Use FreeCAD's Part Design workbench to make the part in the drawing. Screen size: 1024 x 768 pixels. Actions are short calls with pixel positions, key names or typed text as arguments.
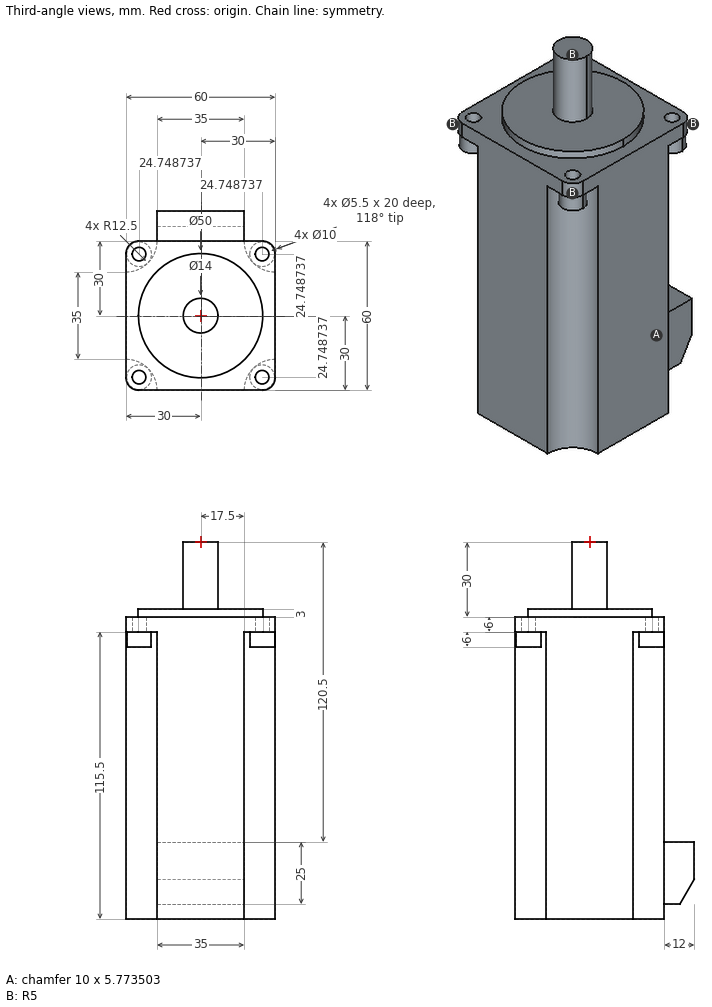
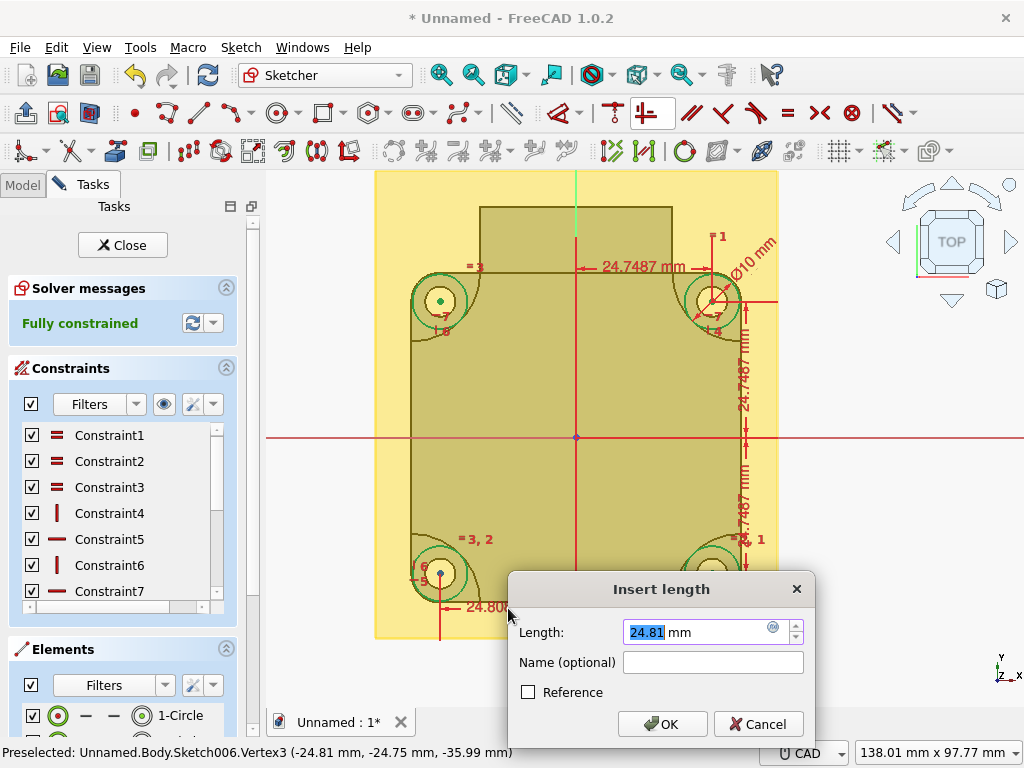
text(24.748737)
key(Return)
key(Escape)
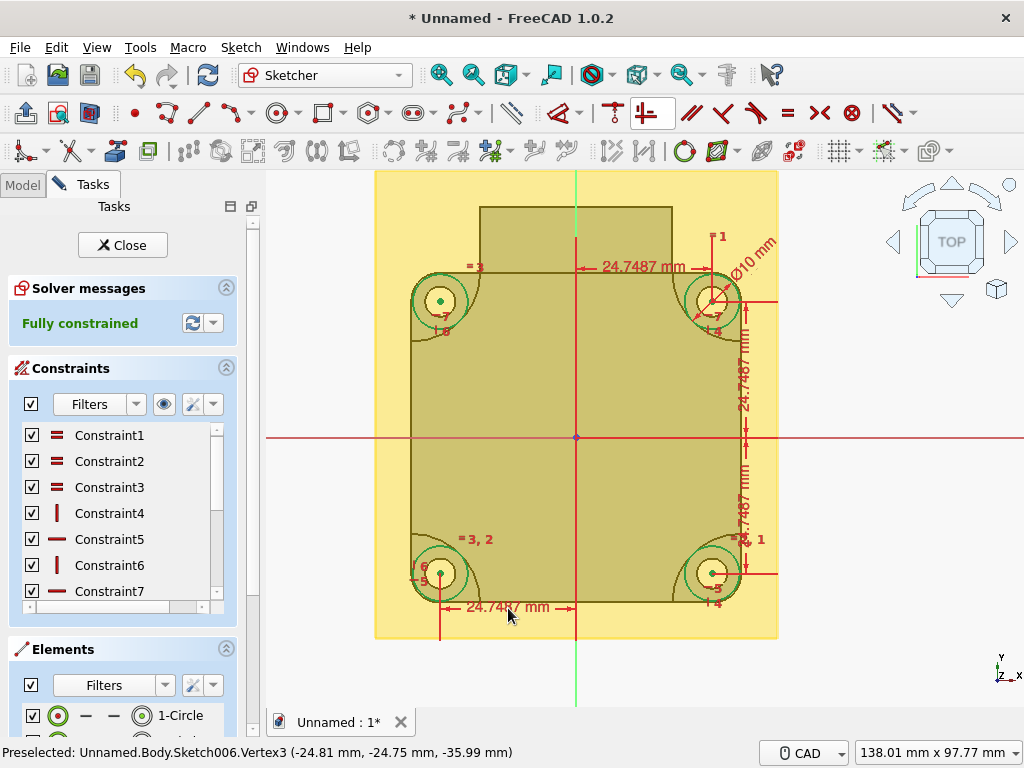
click(123, 245)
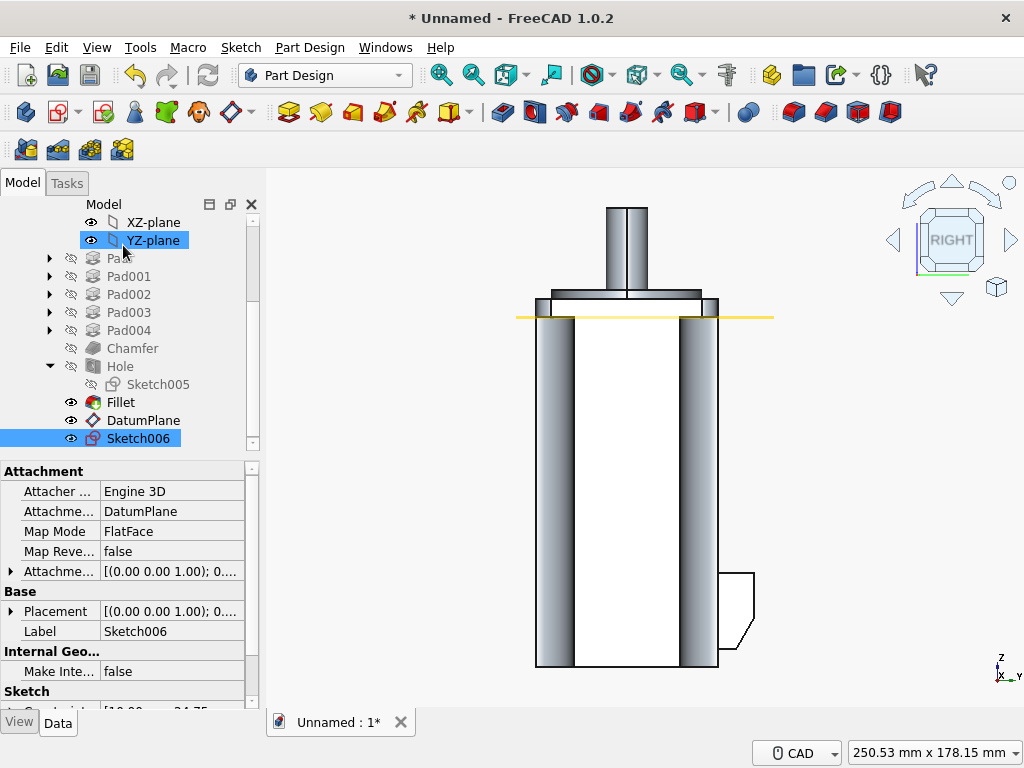
click(290, 112)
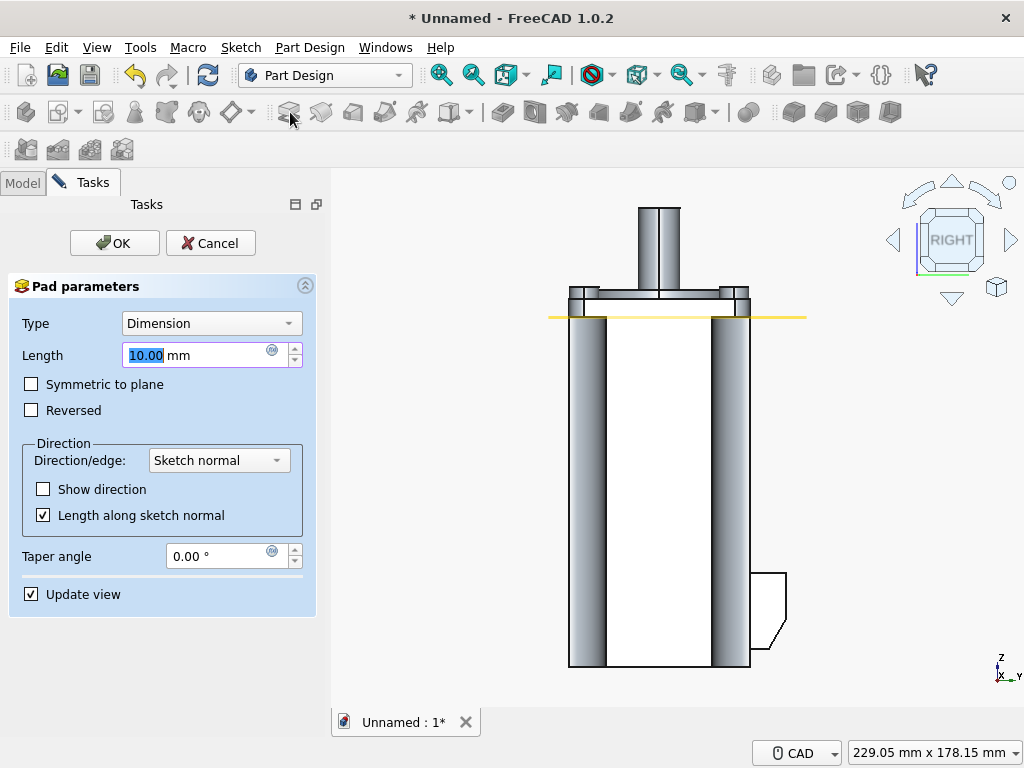
text(6)
key(Tab)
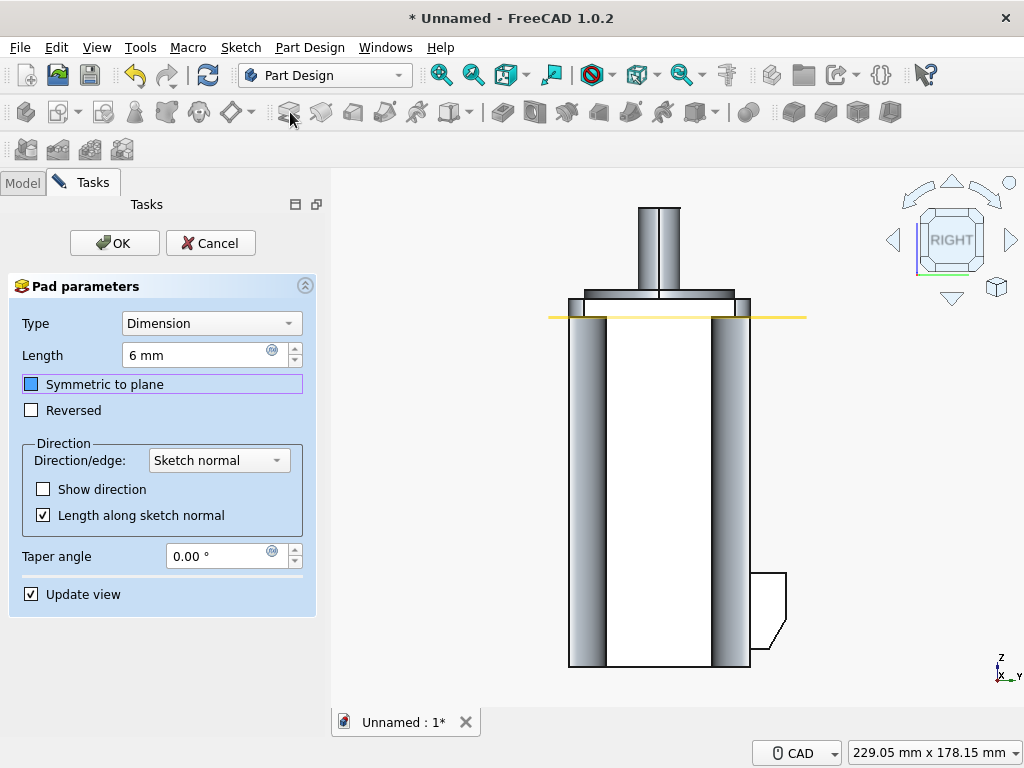
click(30, 410)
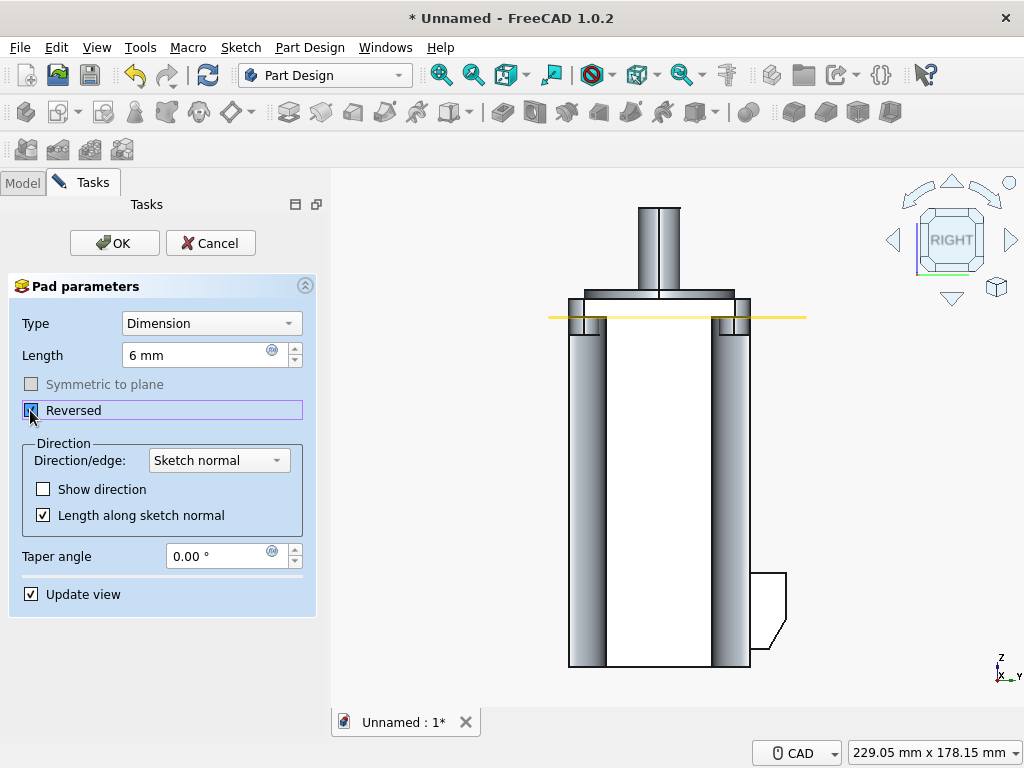
click(115, 243)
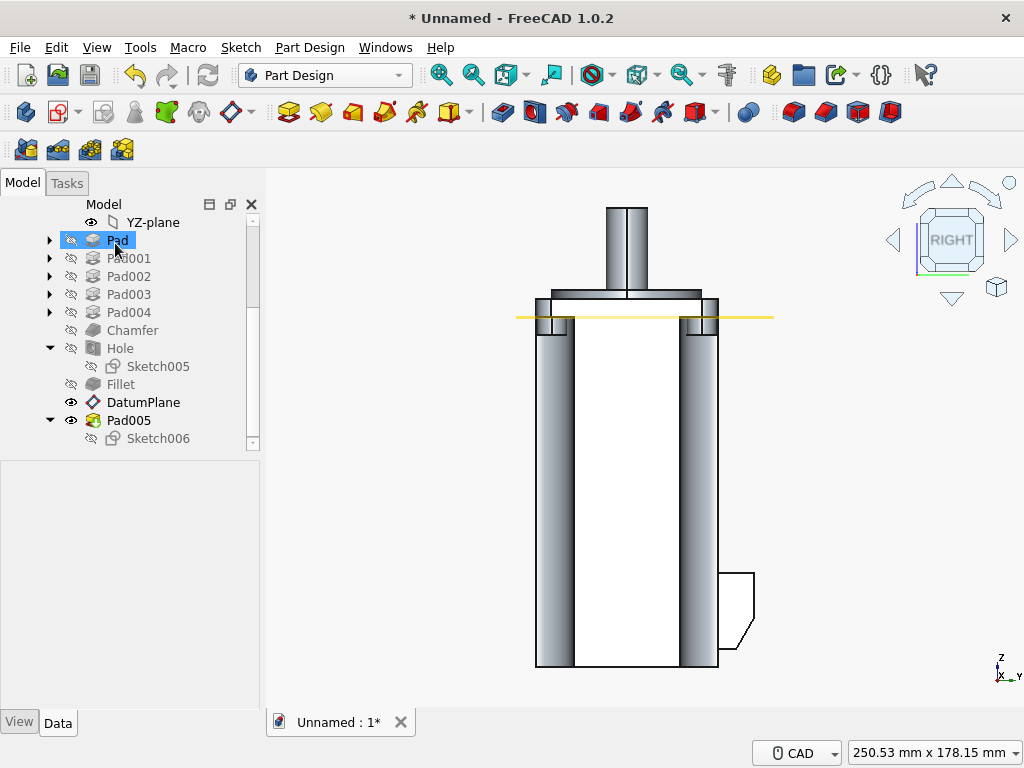
click(116, 402)
key(space)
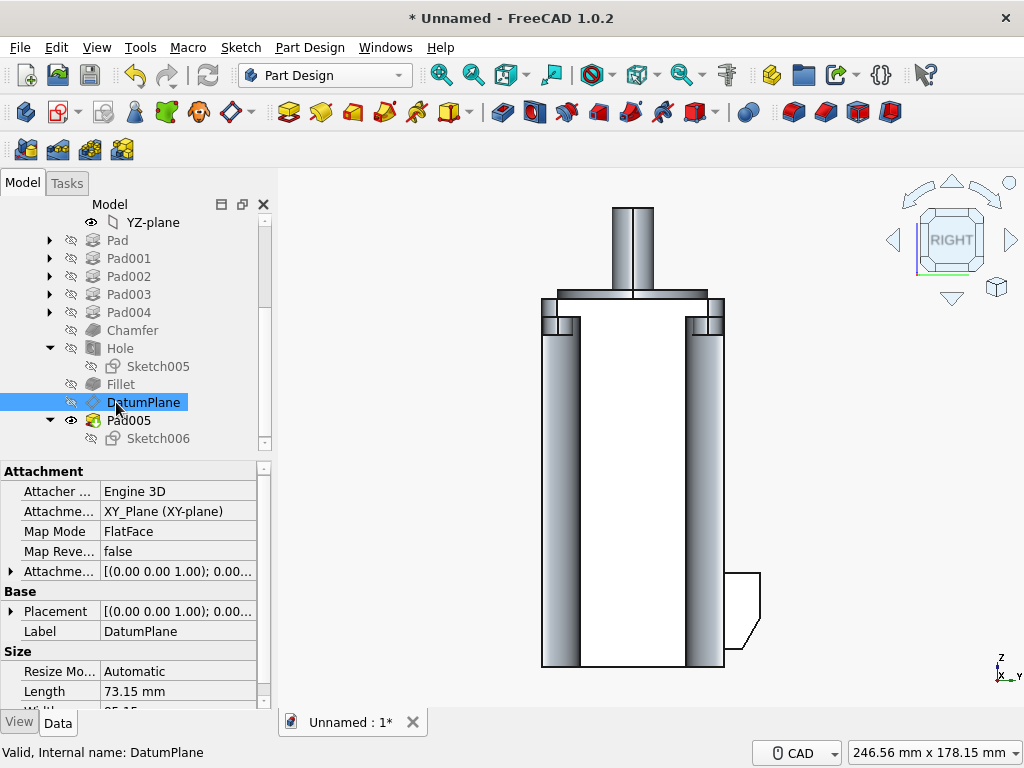
key(0)